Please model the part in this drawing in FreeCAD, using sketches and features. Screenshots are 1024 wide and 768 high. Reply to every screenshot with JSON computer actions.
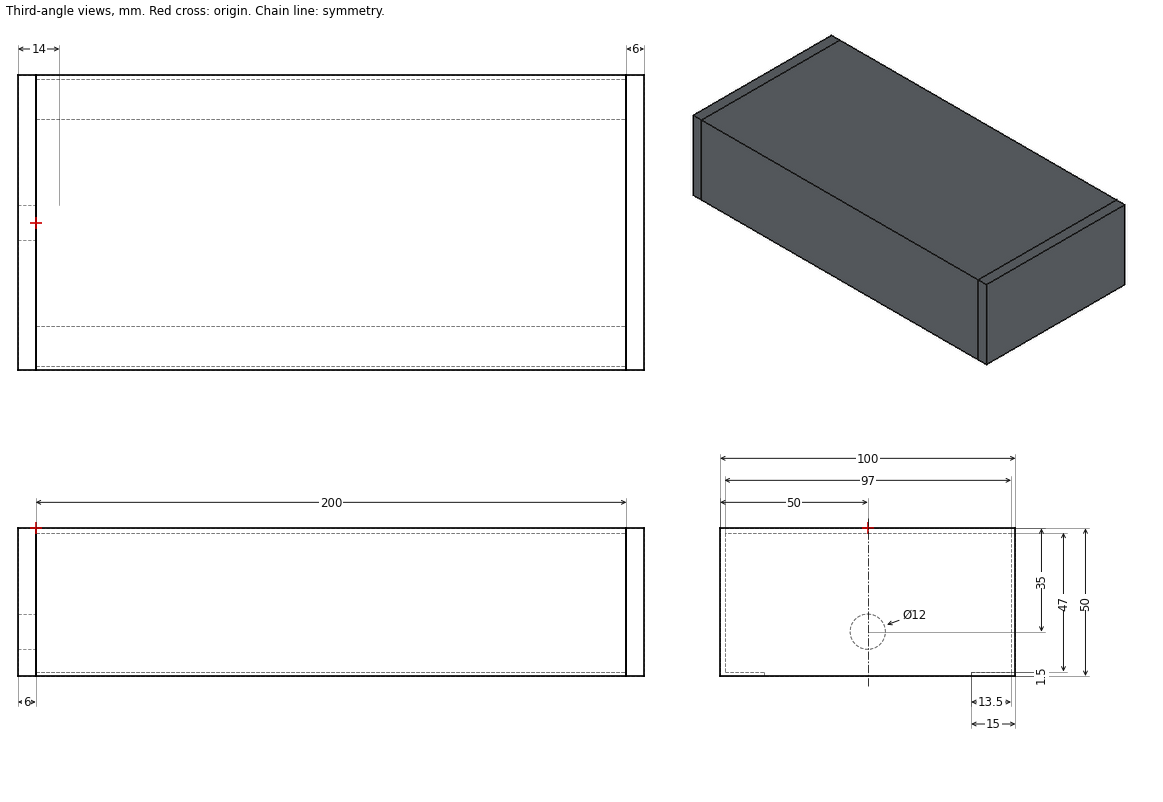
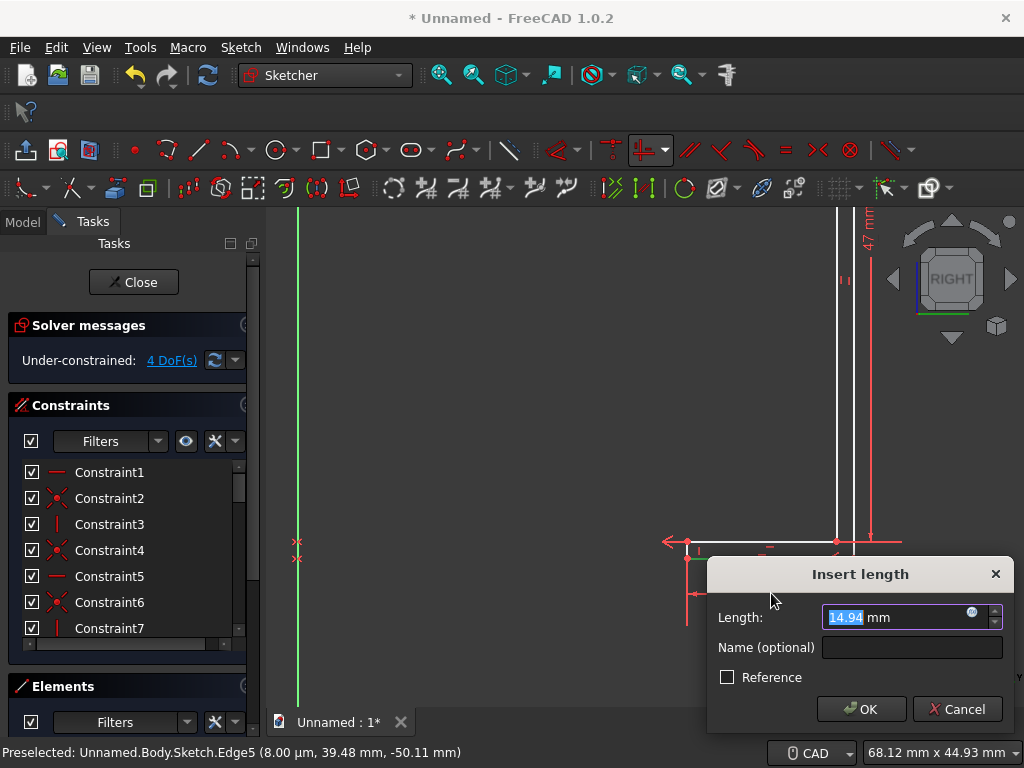
{"action": "type", "text": "15"}
{"action": "key", "text": "Return"}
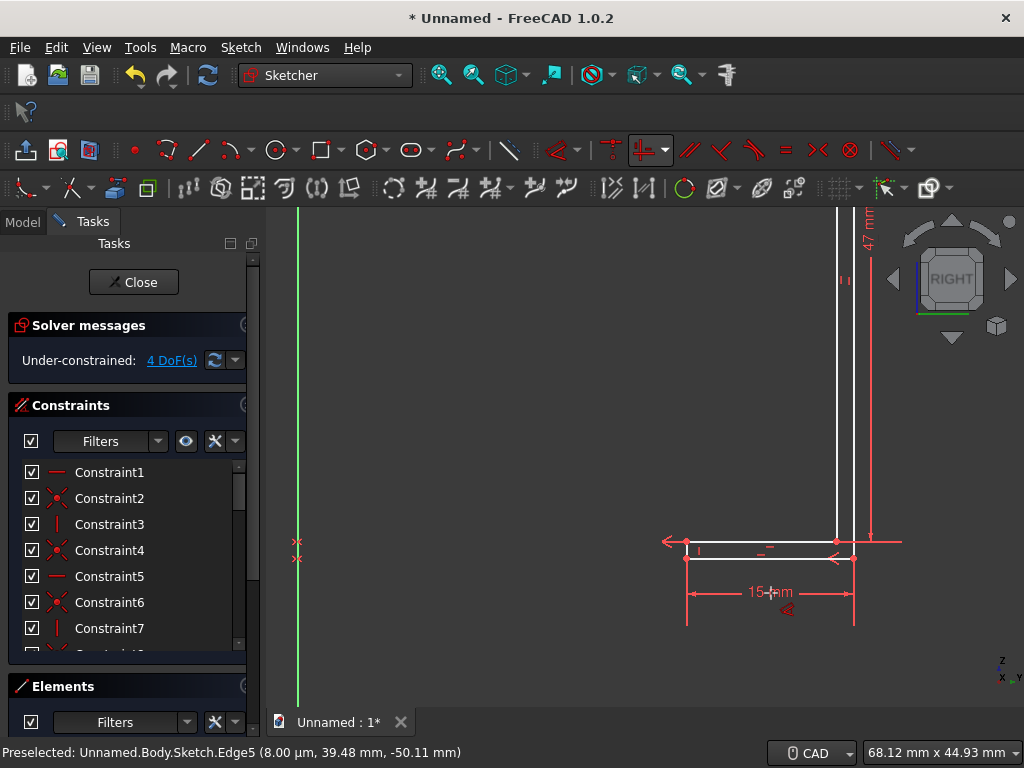
{"action": "left_click", "coordinate": [854, 391]}
{"action": "left_click", "coordinate": [820, 397]}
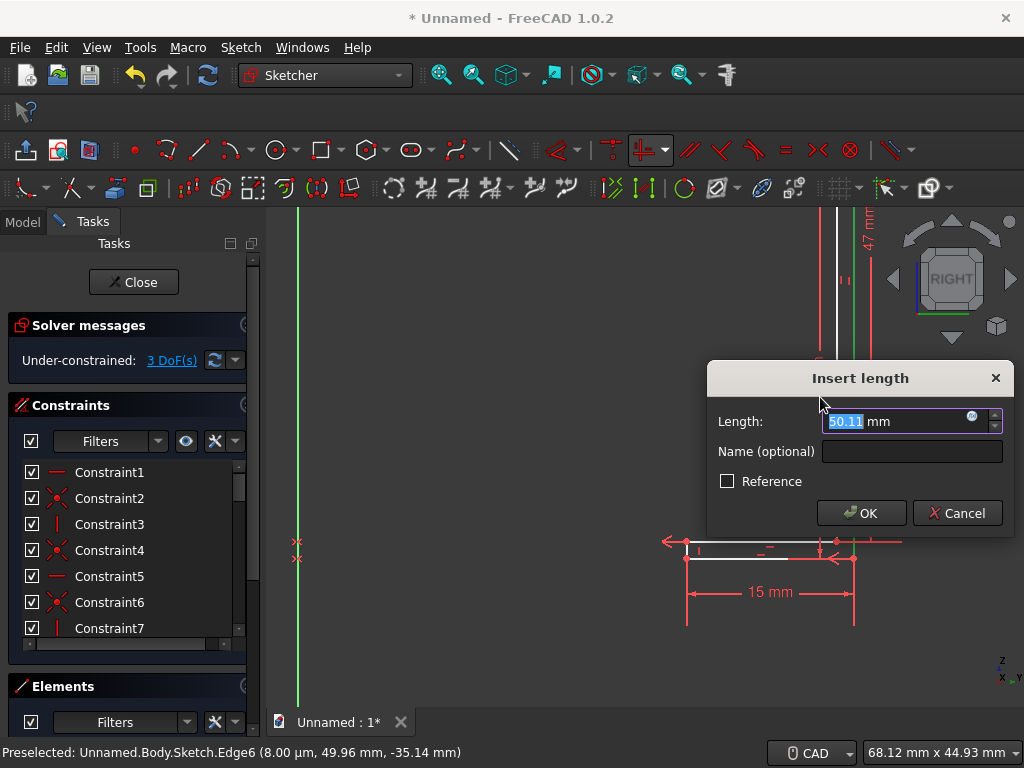
{"action": "type", "text": "50"}
{"action": "key", "text": "Return"}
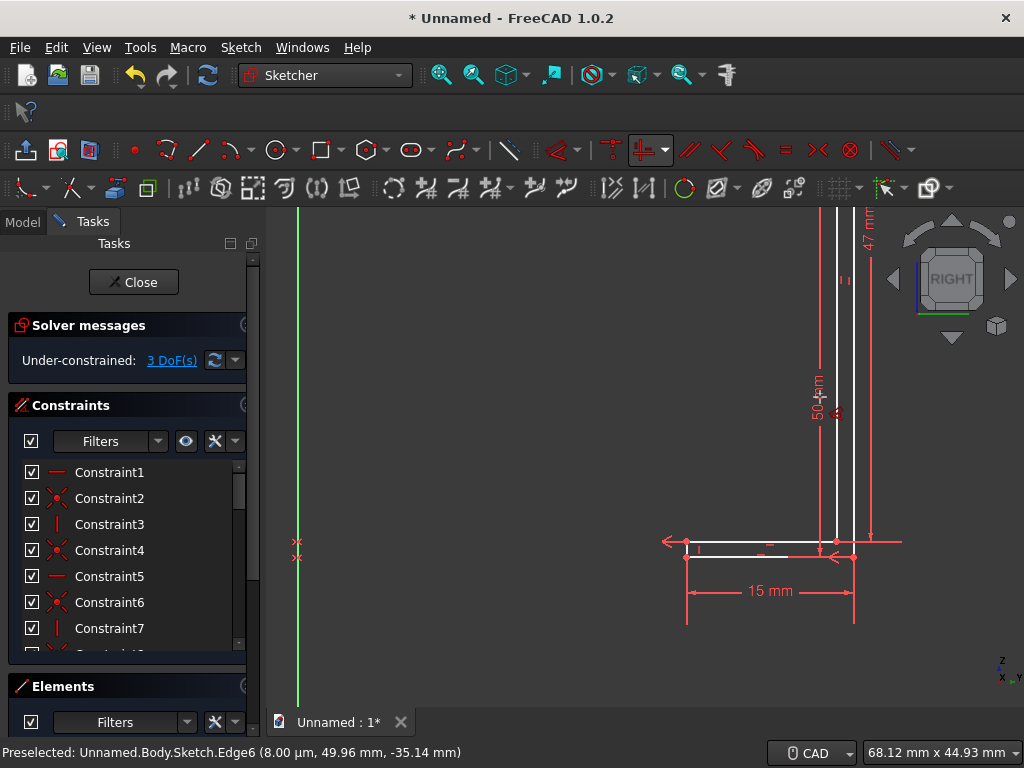
{"action": "scroll", "coordinate": [687, 550], "scroll_direction": "up", "scroll_amount": 5}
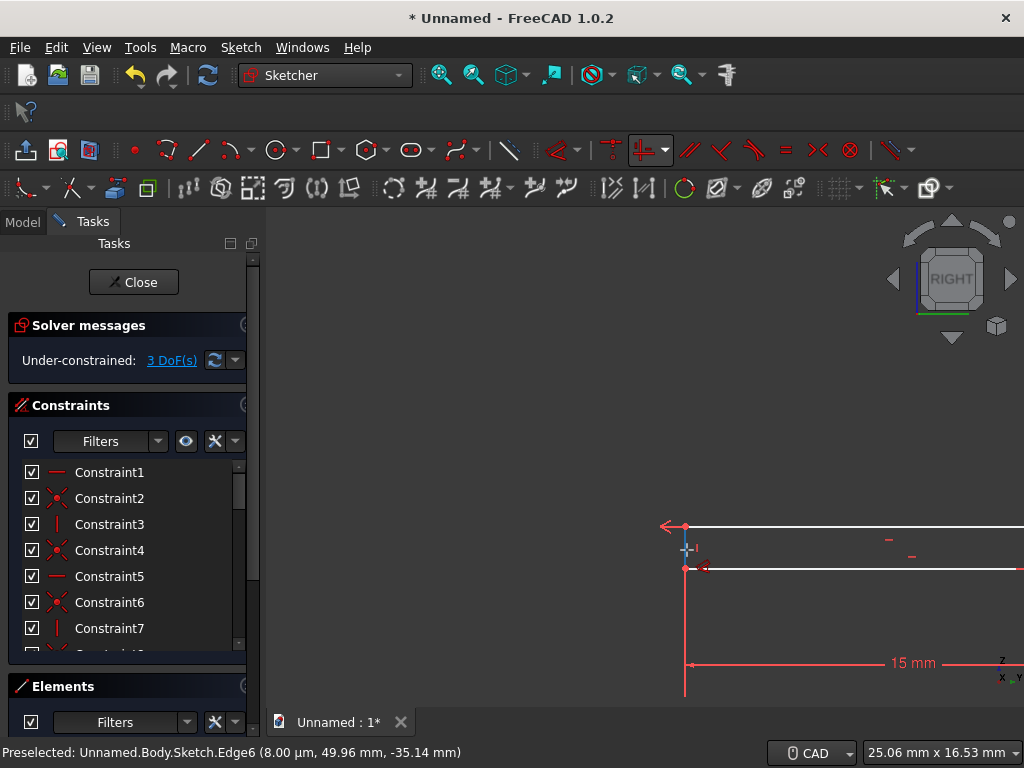
{"action": "left_click", "coordinate": [685, 548]}
{"action": "left_click", "coordinate": [719, 548]}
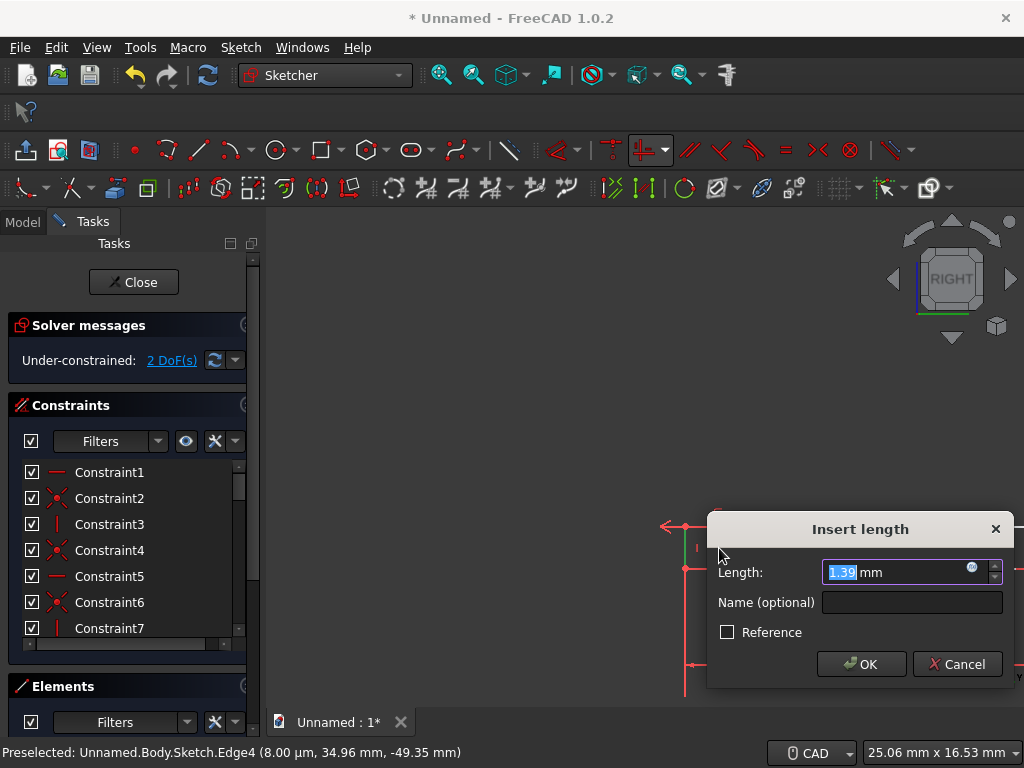
{"action": "type", "text": "1.5"}
{"action": "key", "text": "Return"}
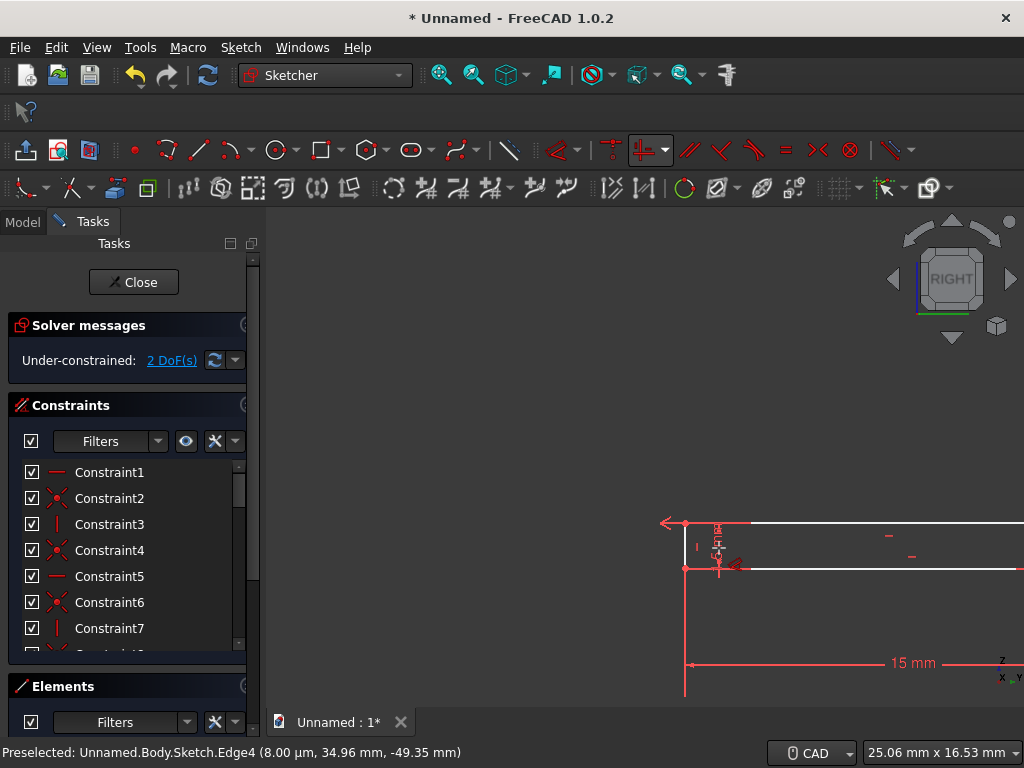
{"action": "scroll", "coordinate": [725, 558], "scroll_direction": "down", "scroll_amount": 10}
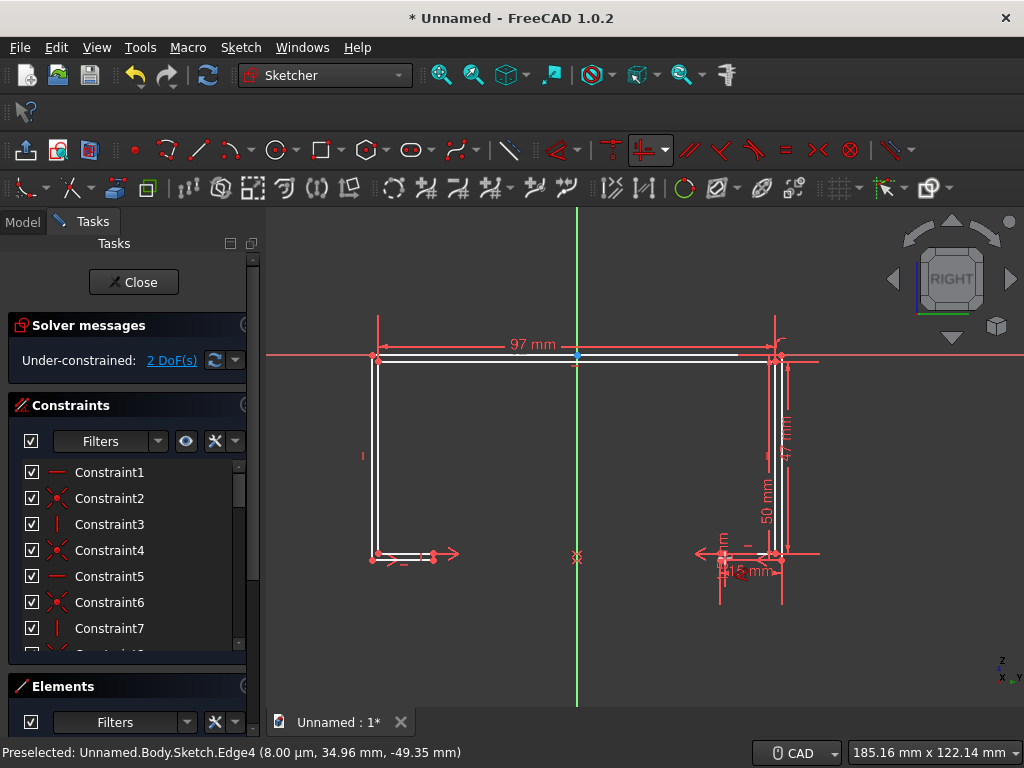
{"action": "scroll", "coordinate": [659, 355], "scroll_direction": "up", "scroll_amount": 5}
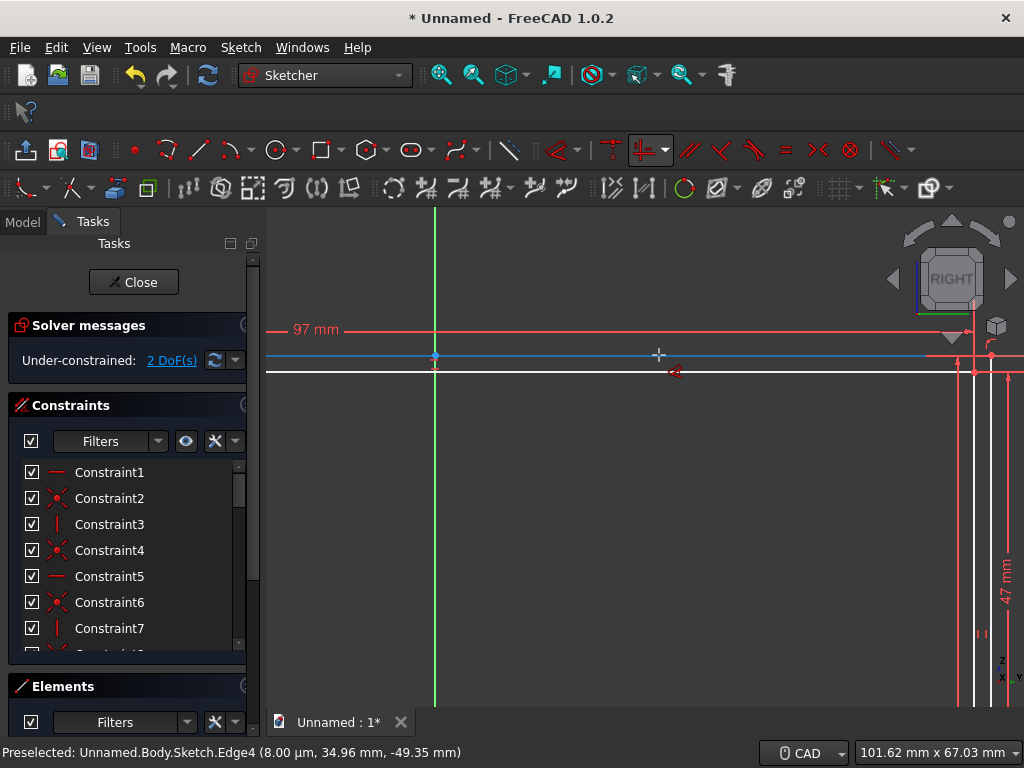
{"action": "left_click", "coordinate": [658, 356]}
{"action": "left_click", "coordinate": [576, 322]}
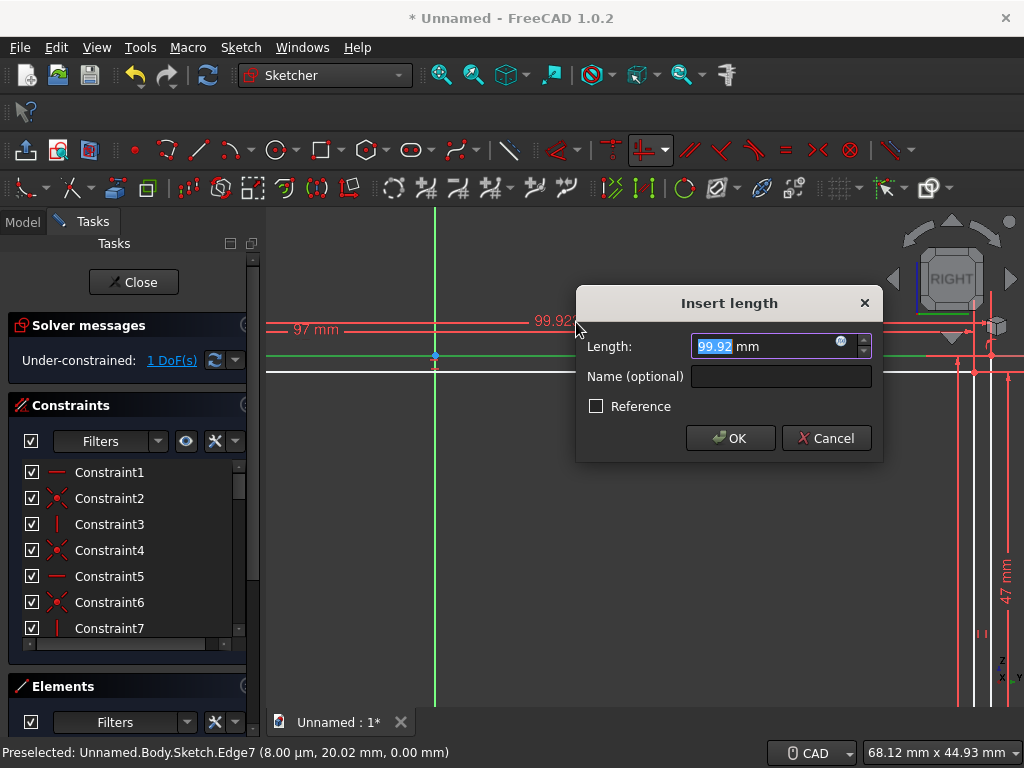
{"action": "type", "text": "100"}
{"action": "key", "text": "Return"}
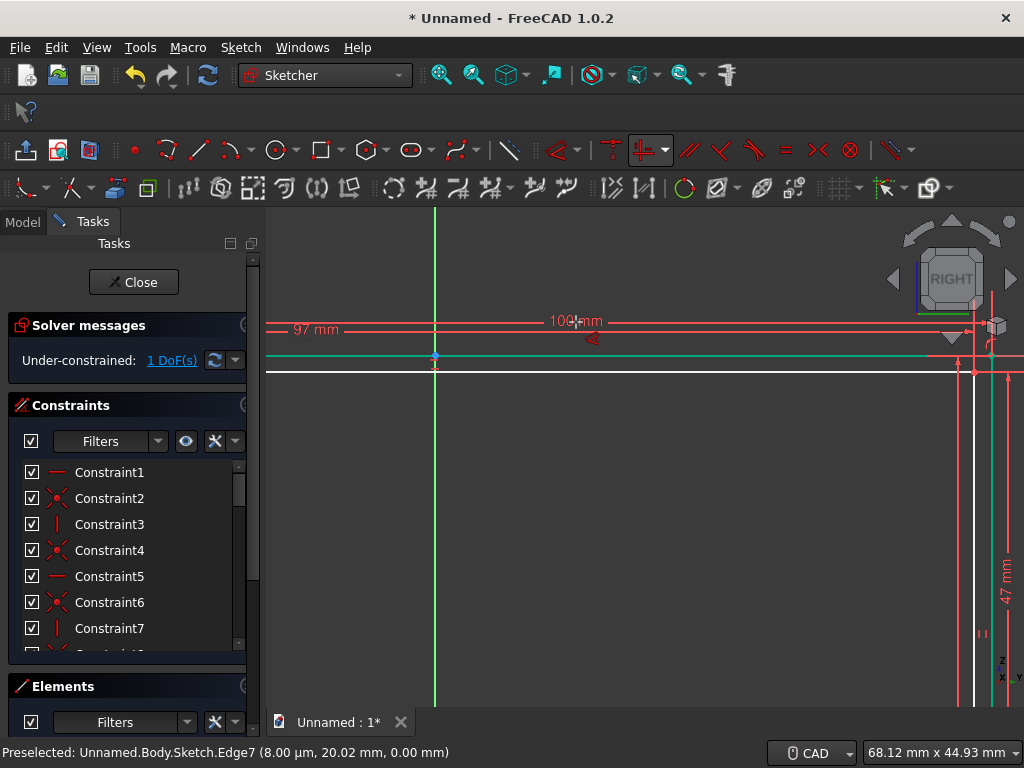
{"action": "scroll", "coordinate": [659, 354], "scroll_direction": "down", "scroll_amount": 5}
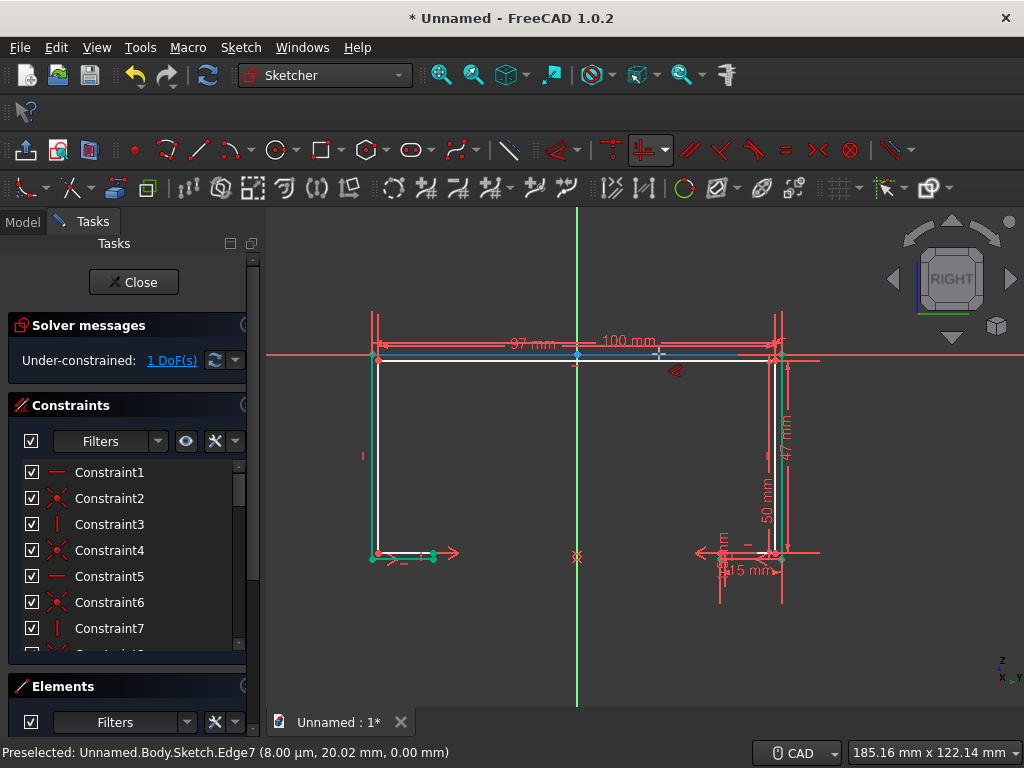
{"action": "scroll", "coordinate": [759, 553], "scroll_direction": "up", "scroll_amount": 5}